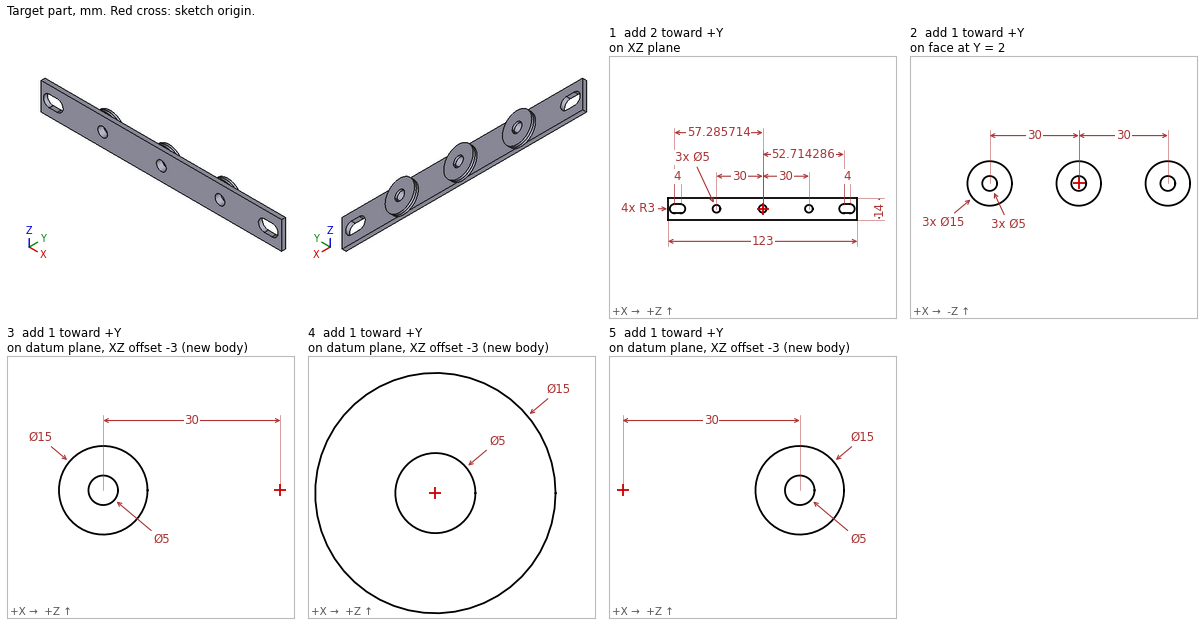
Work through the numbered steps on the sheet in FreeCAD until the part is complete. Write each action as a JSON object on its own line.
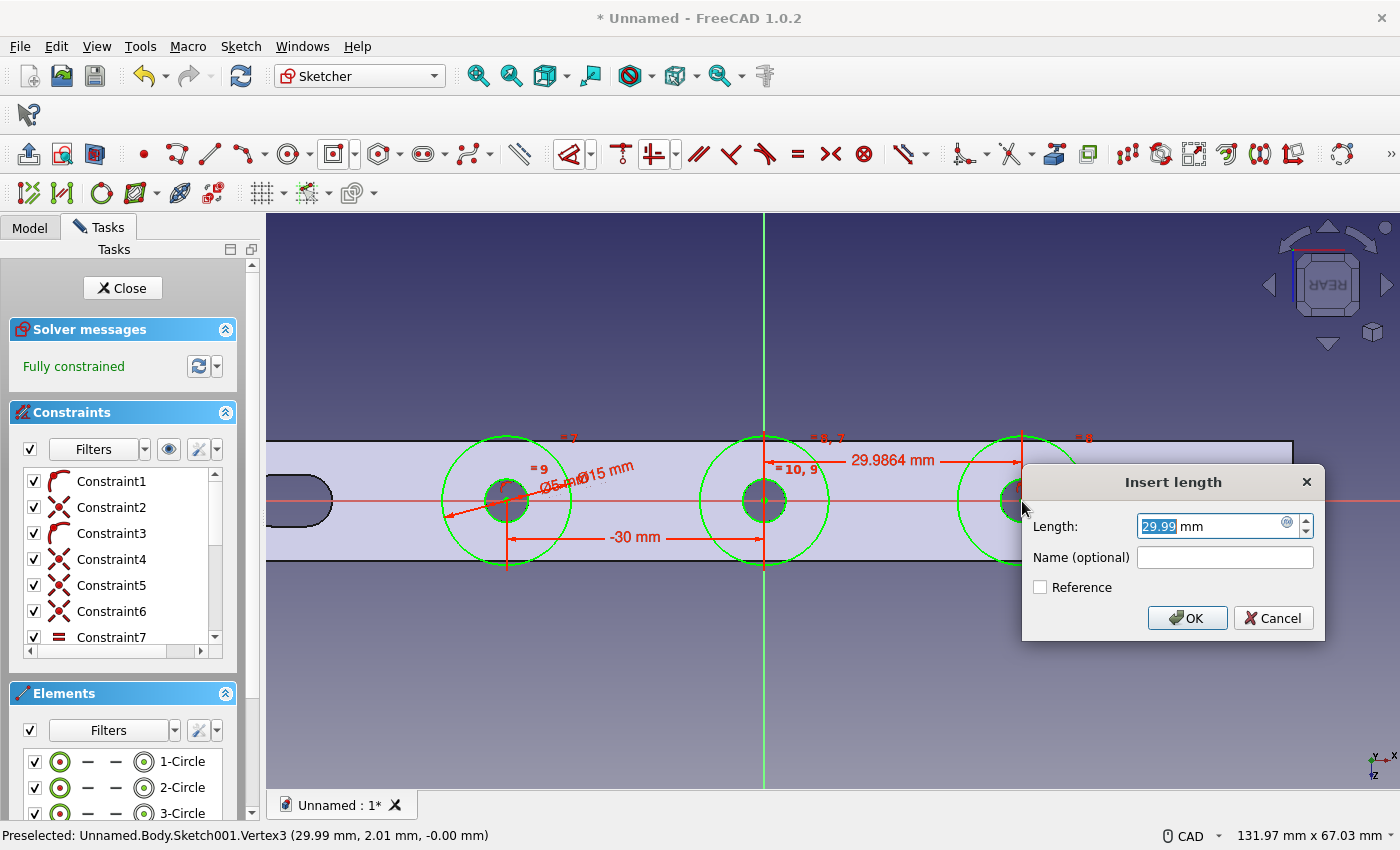
{"action": "type", "text": "30"}
{"action": "key", "text": "Return"}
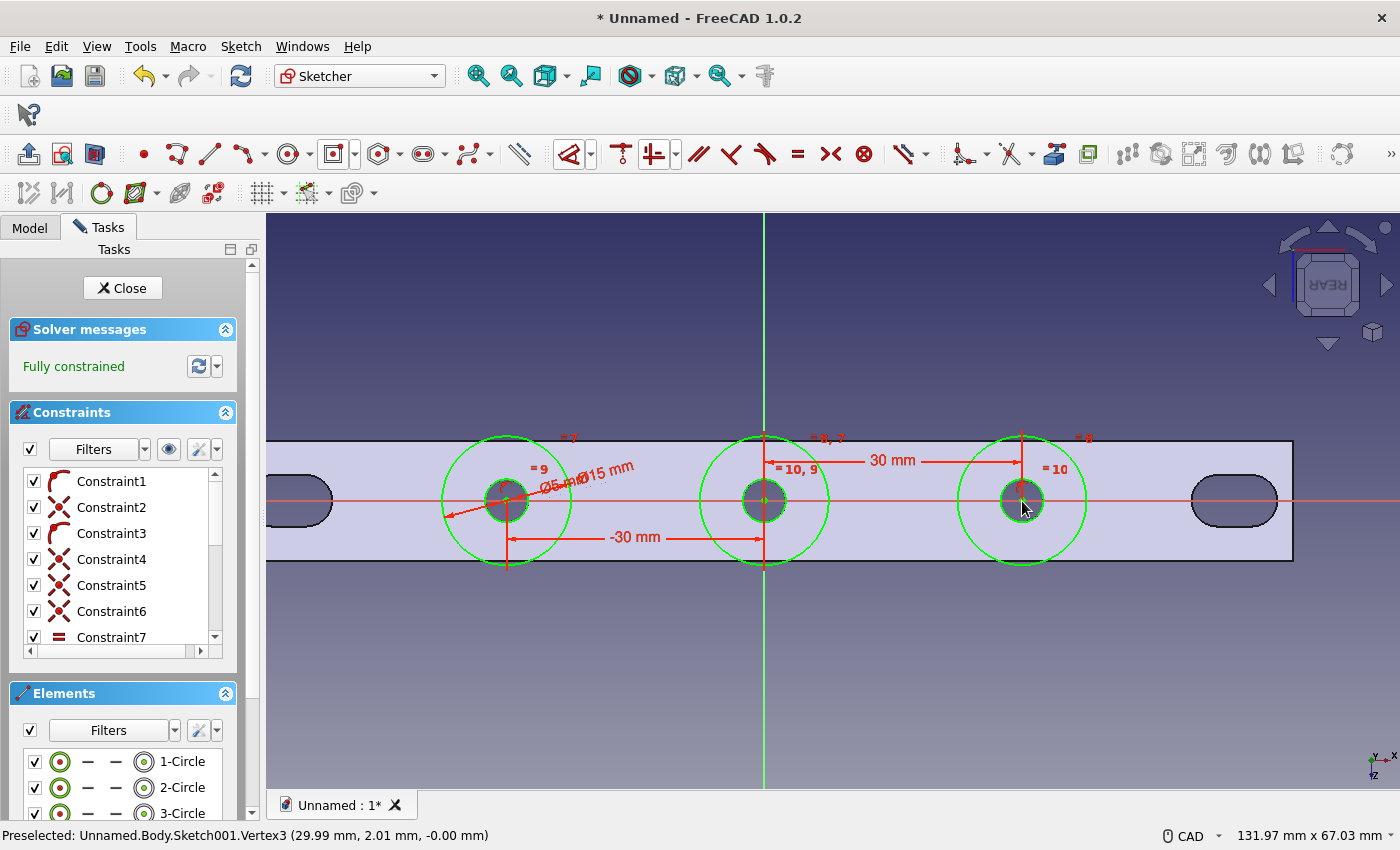
{"action": "left_click", "coordinate": [123, 288]}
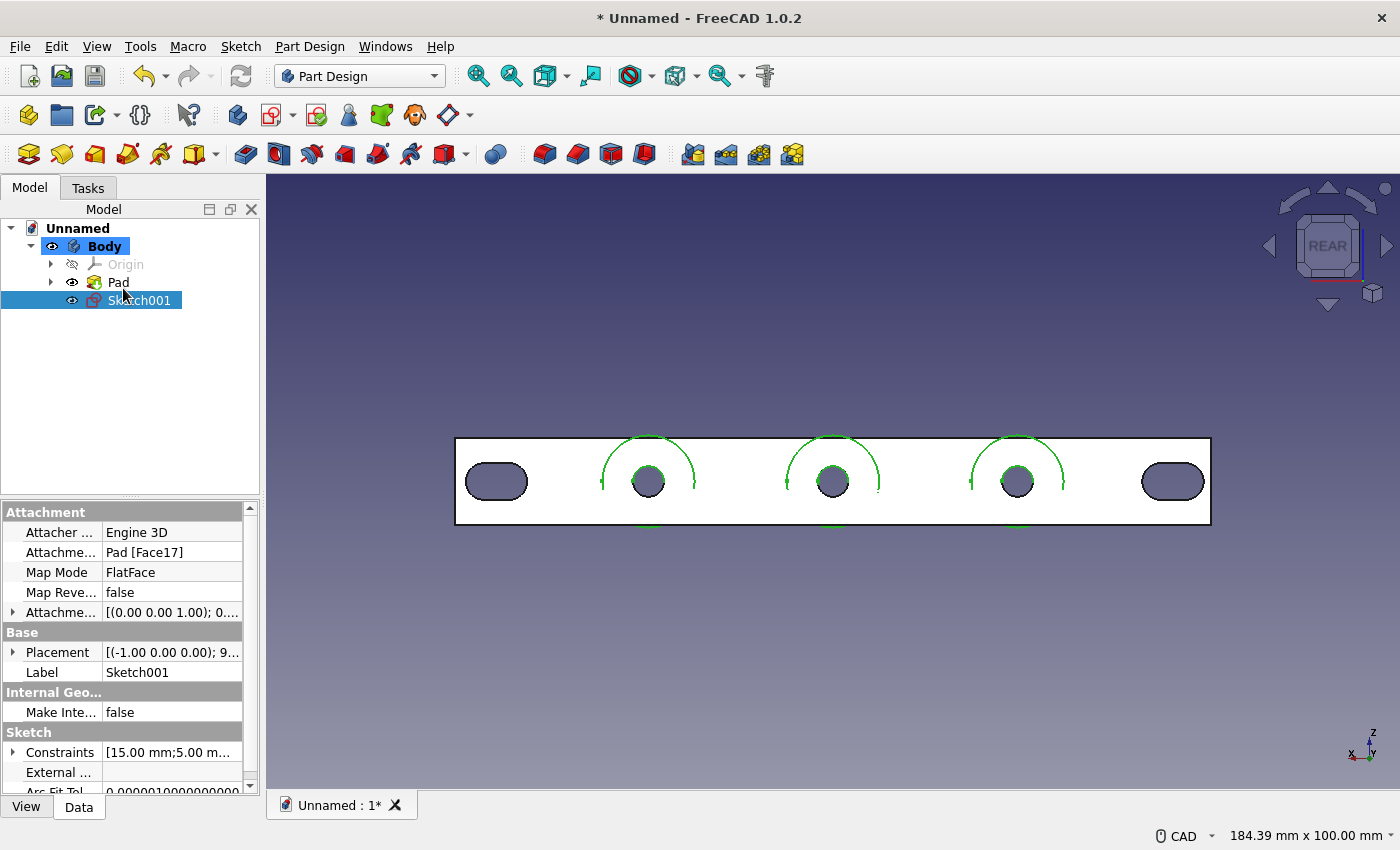
{"action": "left_click", "coordinate": [29, 154]}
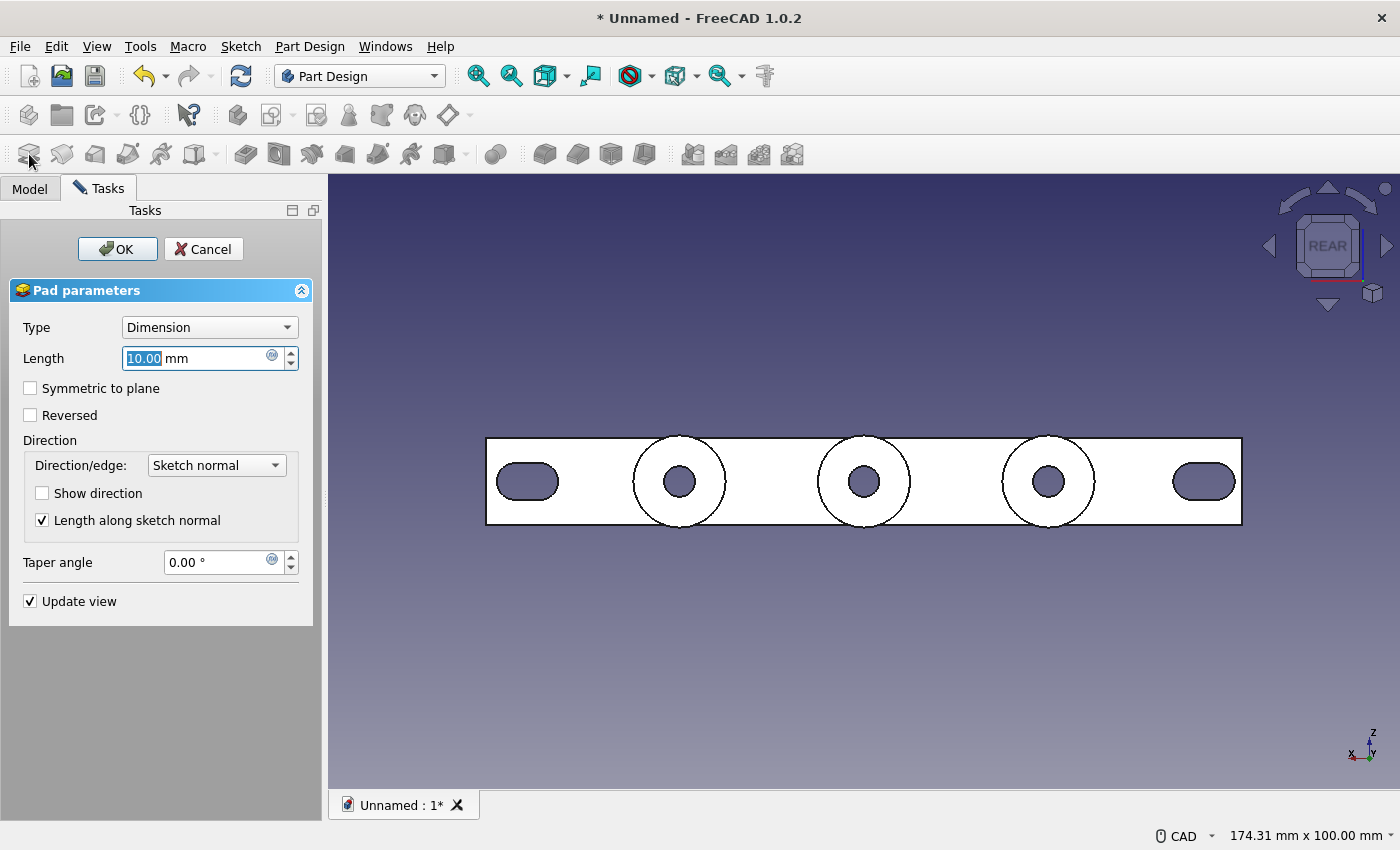
{"action": "type", "text": "1"}
{"action": "key", "text": "Tab"}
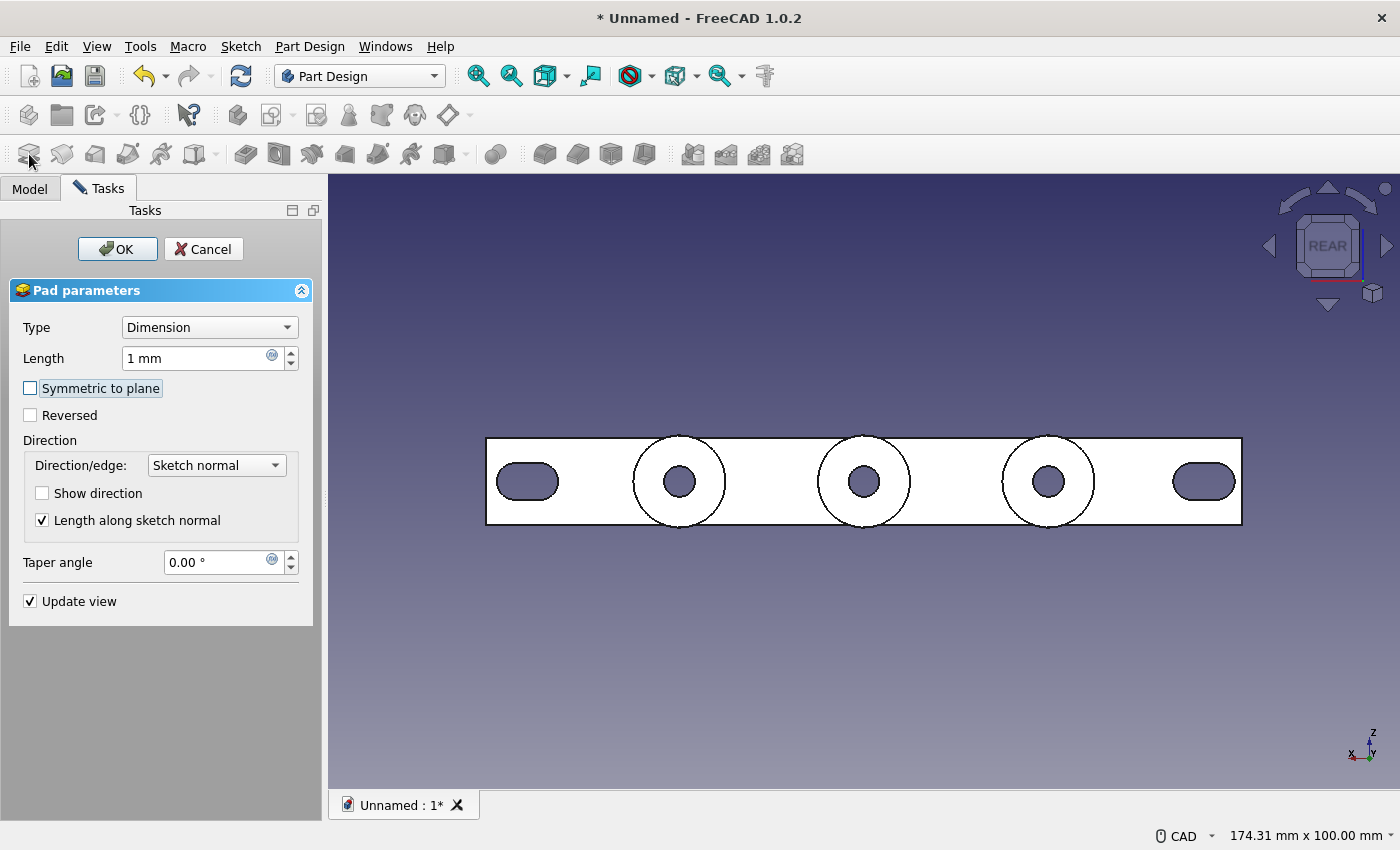
{"action": "left_click", "coordinate": [118, 249]}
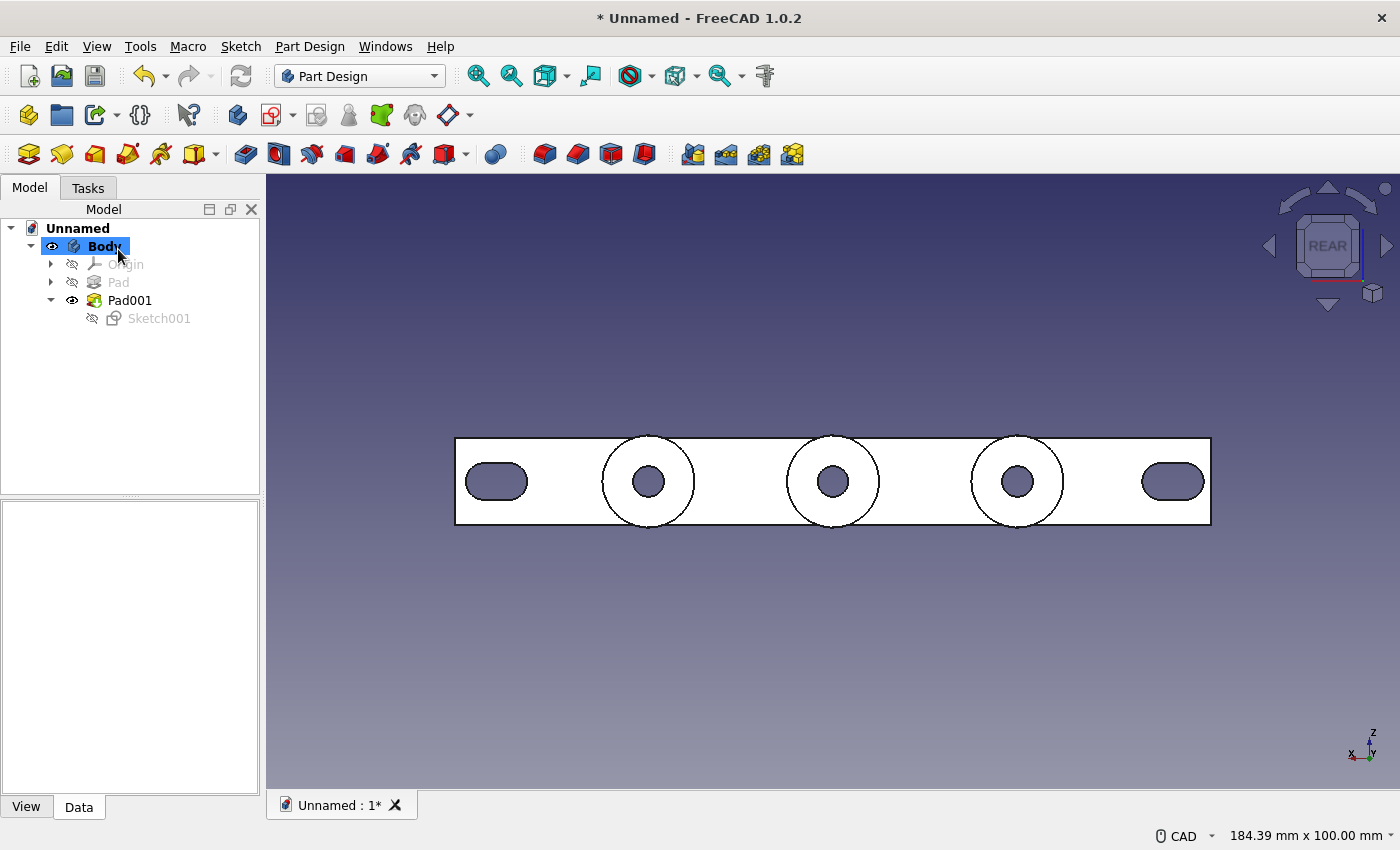
{"action": "left_click", "coordinate": [238, 116]}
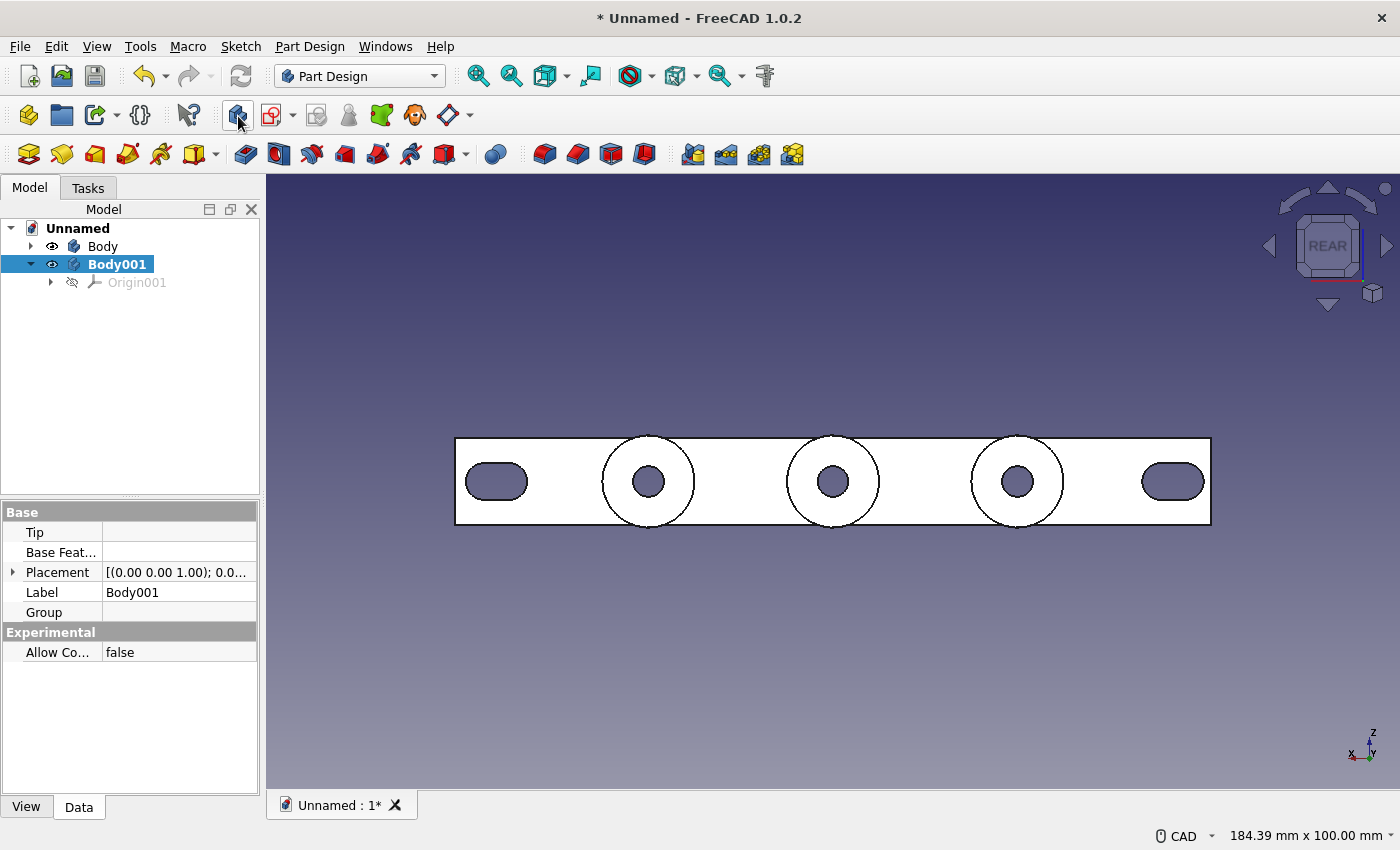
{"action": "left_click", "coordinate": [51, 282]}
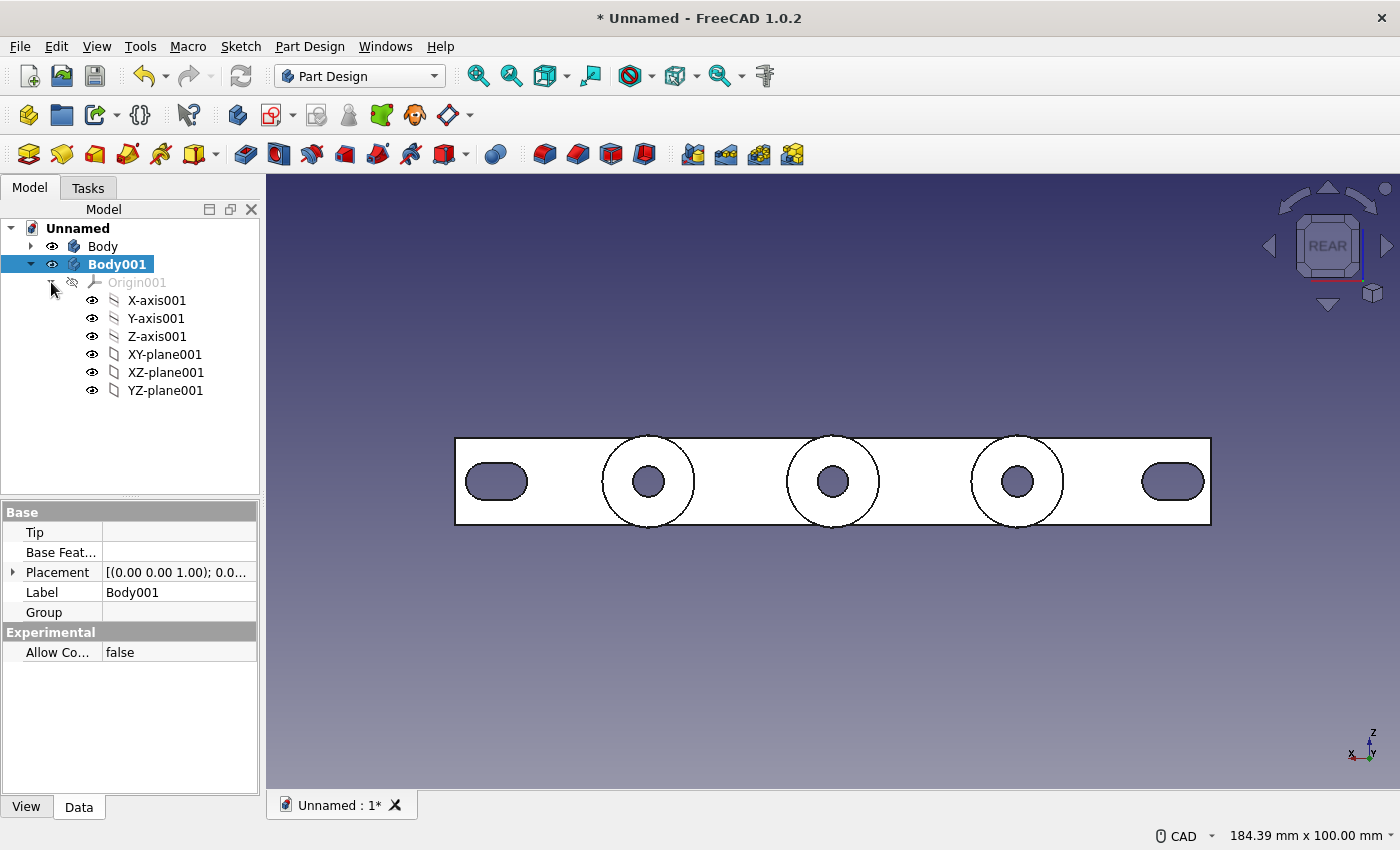
{"action": "left_click", "coordinate": [137, 372]}